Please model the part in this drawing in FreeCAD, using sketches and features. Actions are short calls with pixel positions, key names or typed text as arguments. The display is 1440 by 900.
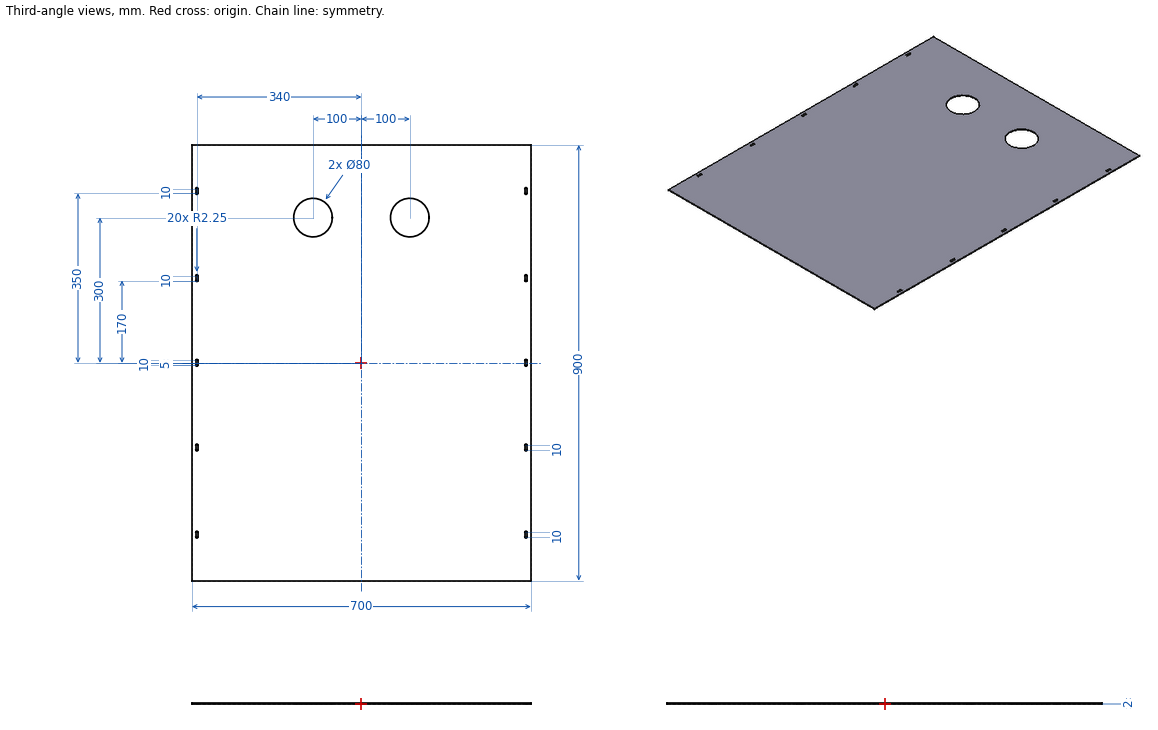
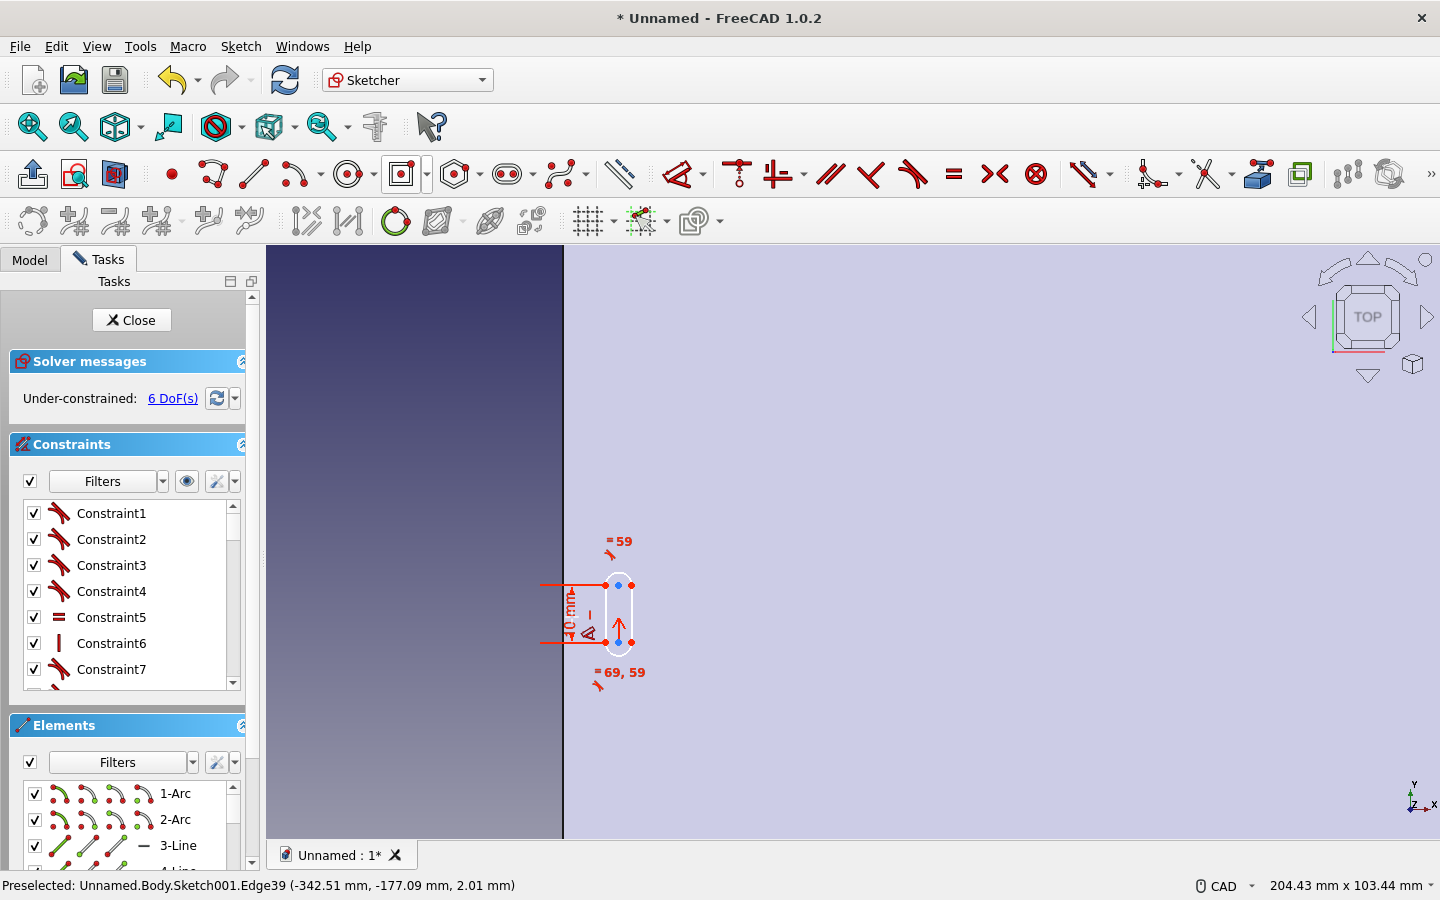
scroll(606, 635, down, 12)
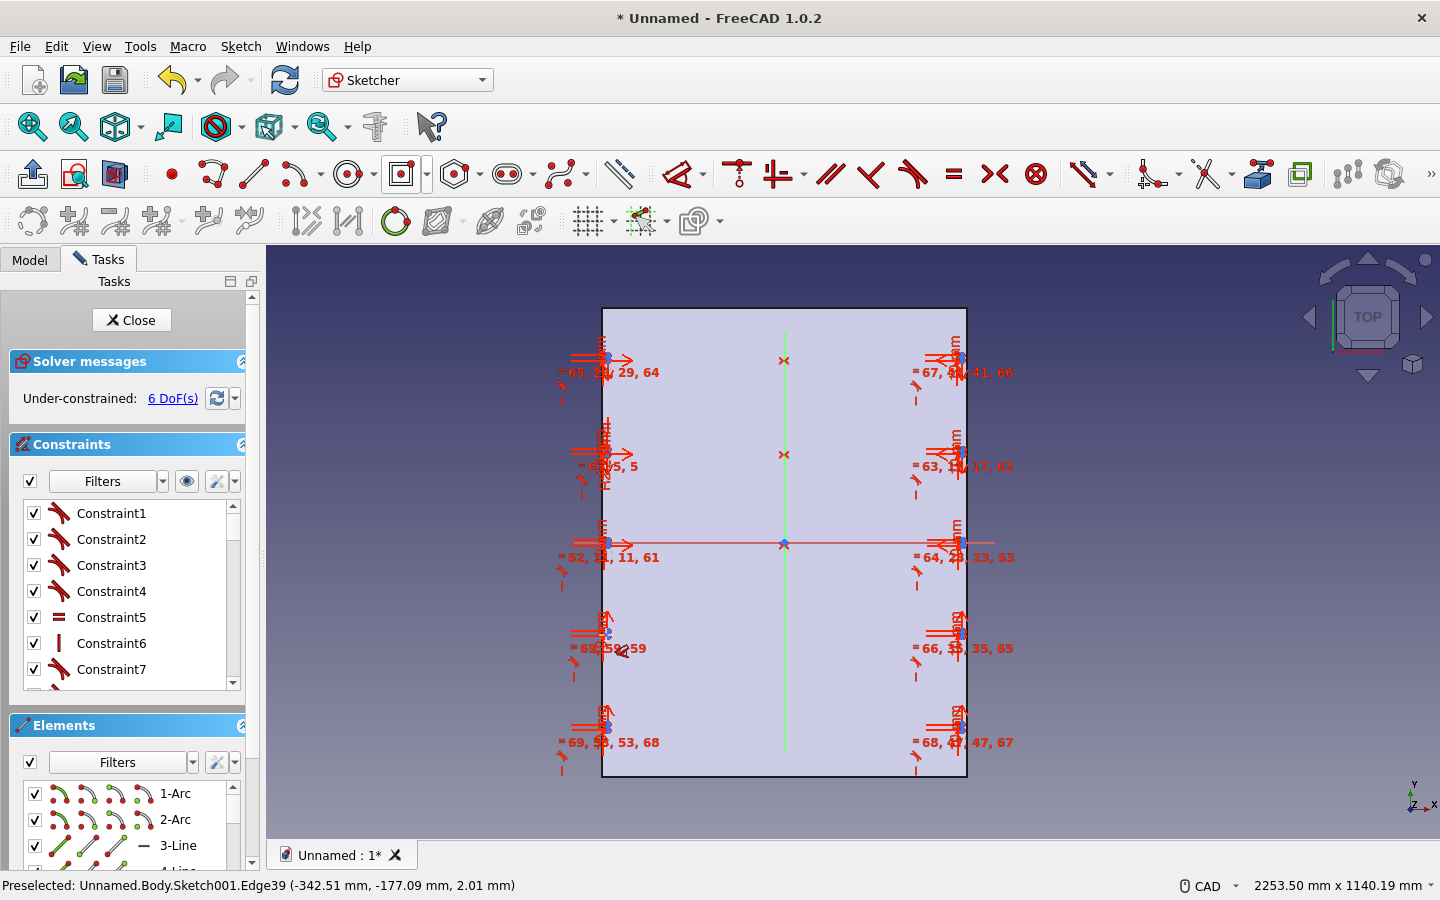
scroll(606, 546, up, 14)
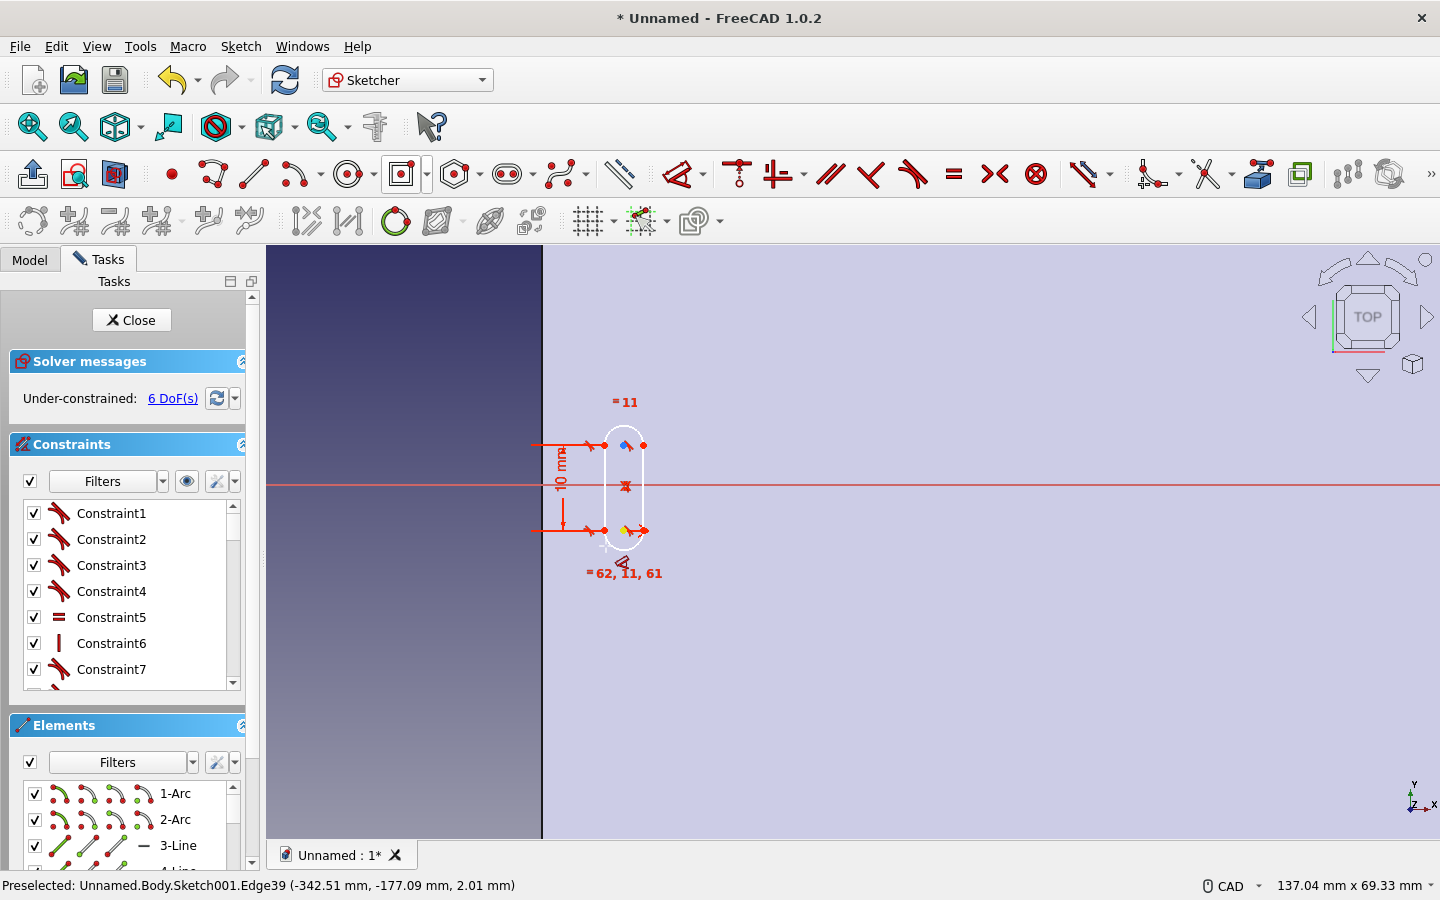
click(605, 531)
click(571, 508)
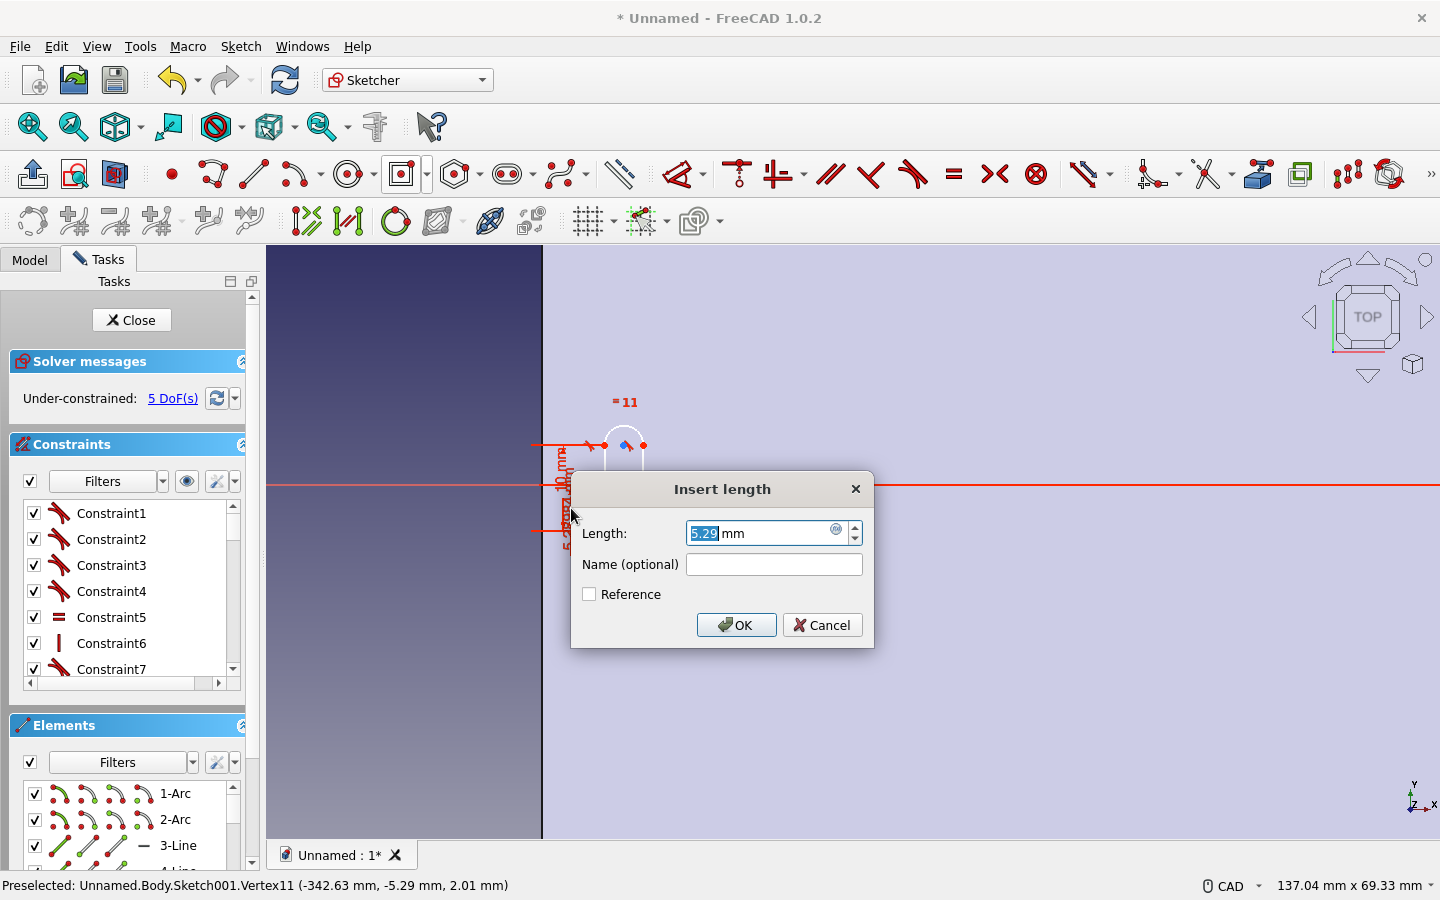
text(5)
key(Return)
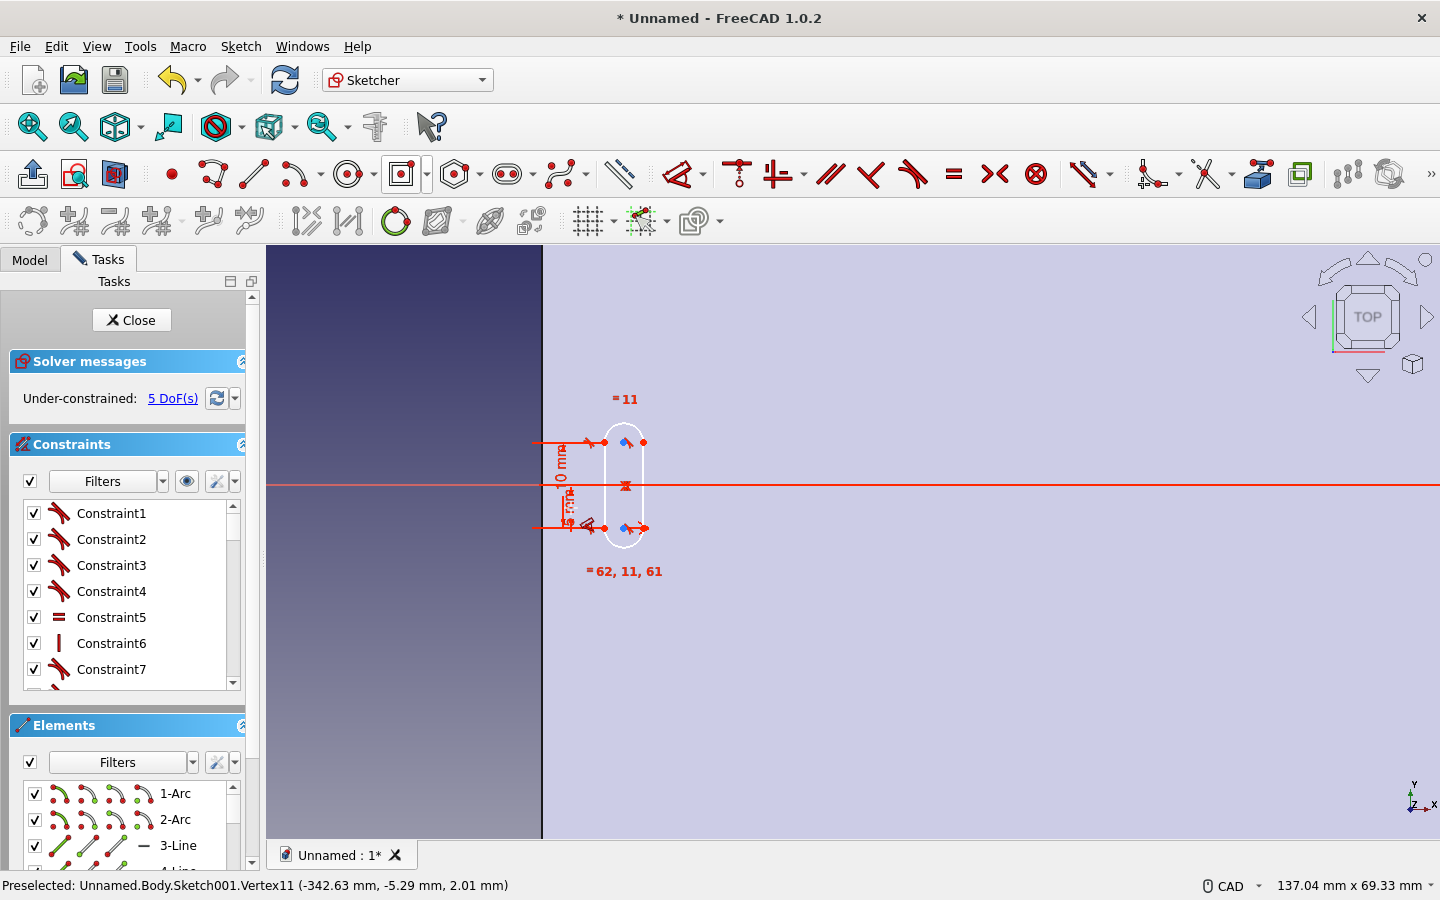
scroll(606, 546, down, 14)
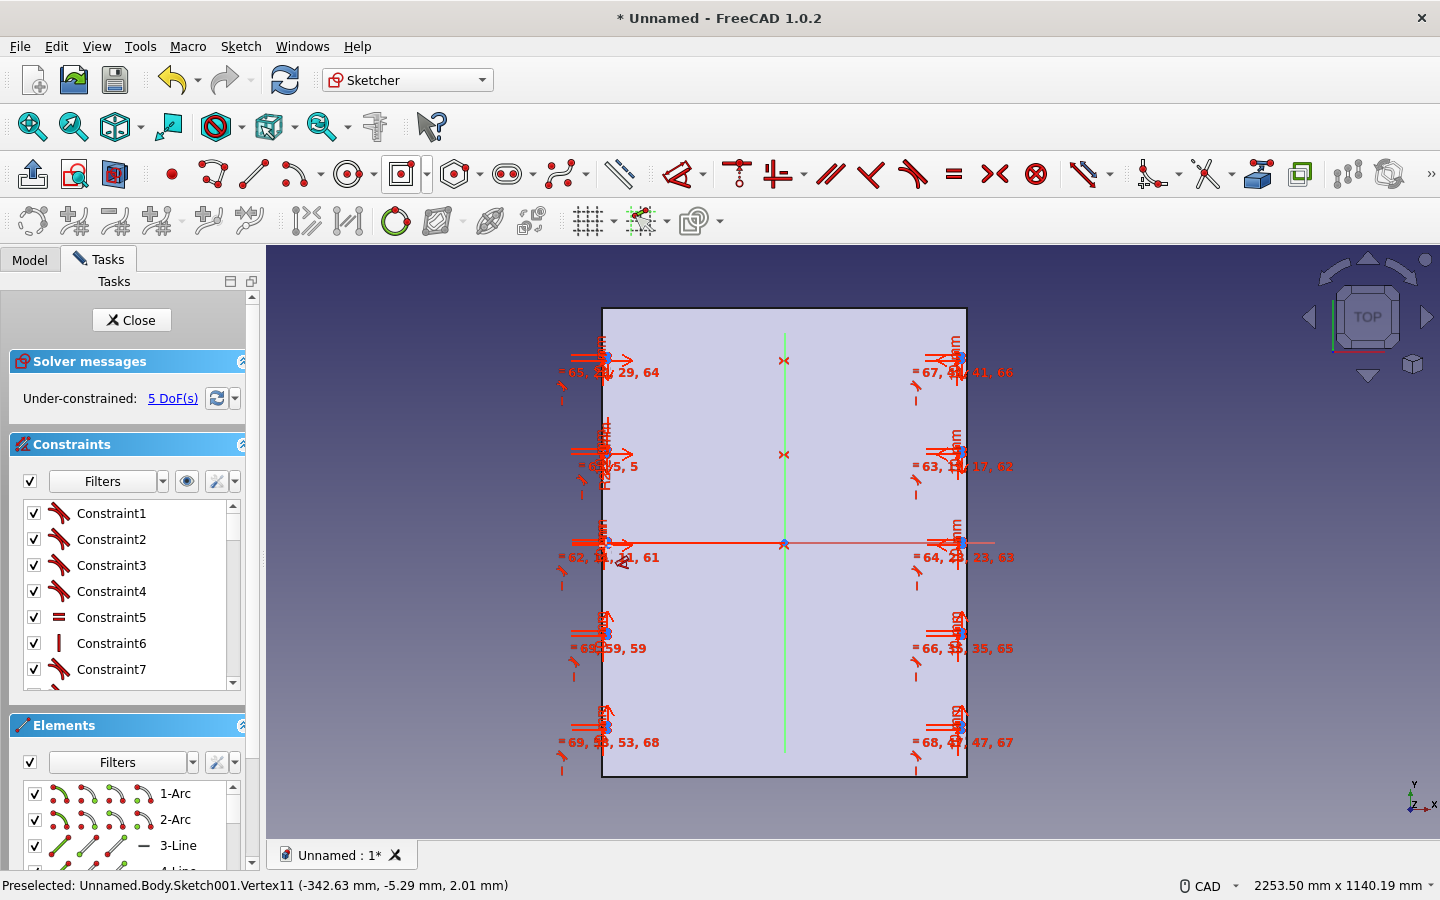
scroll(606, 454, up, 12)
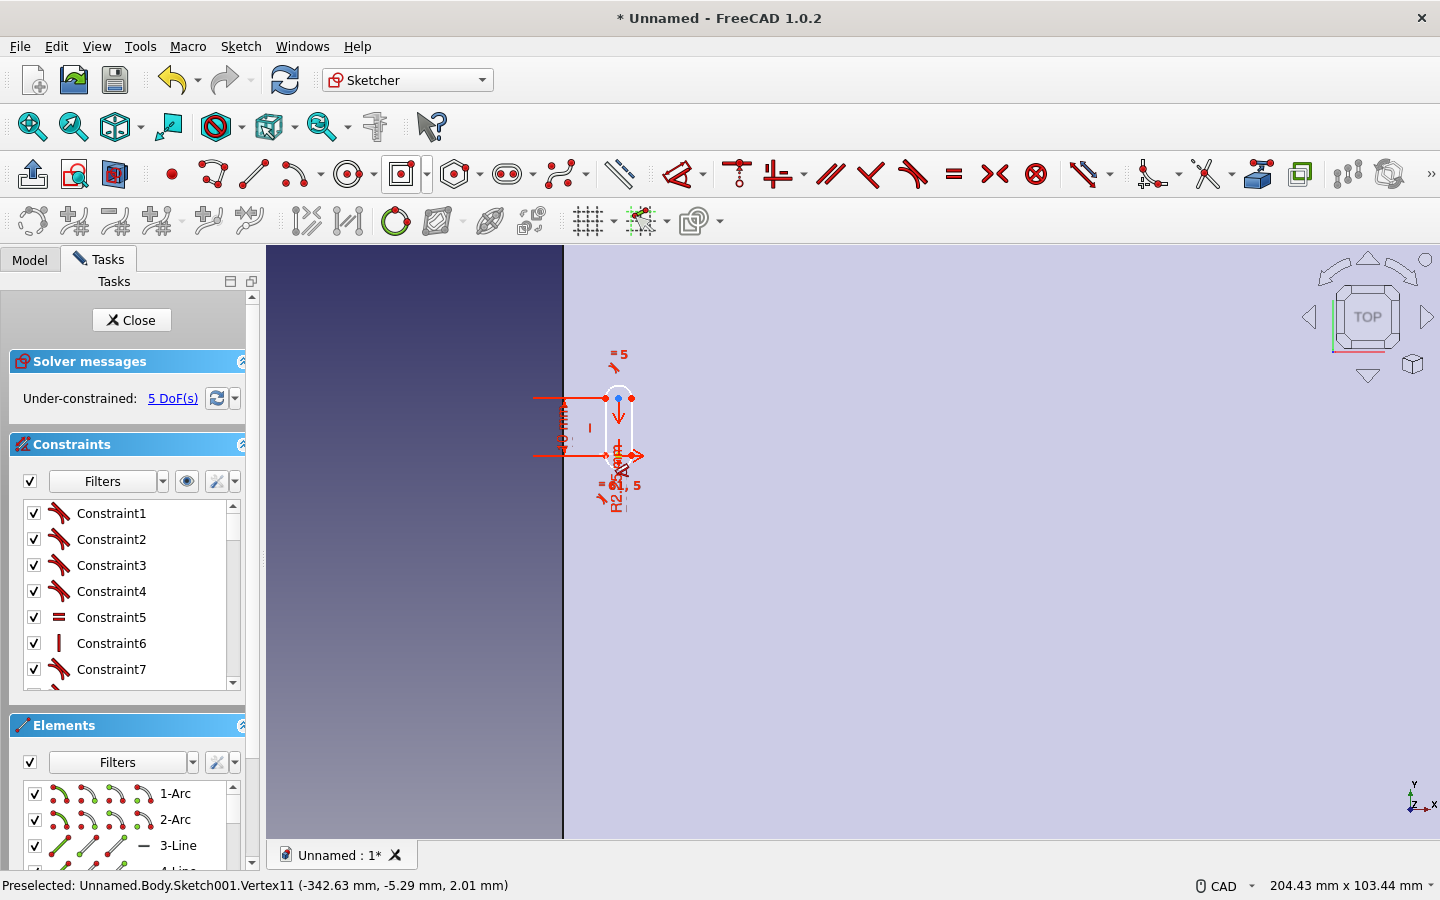
click(606, 456)
click(572, 633)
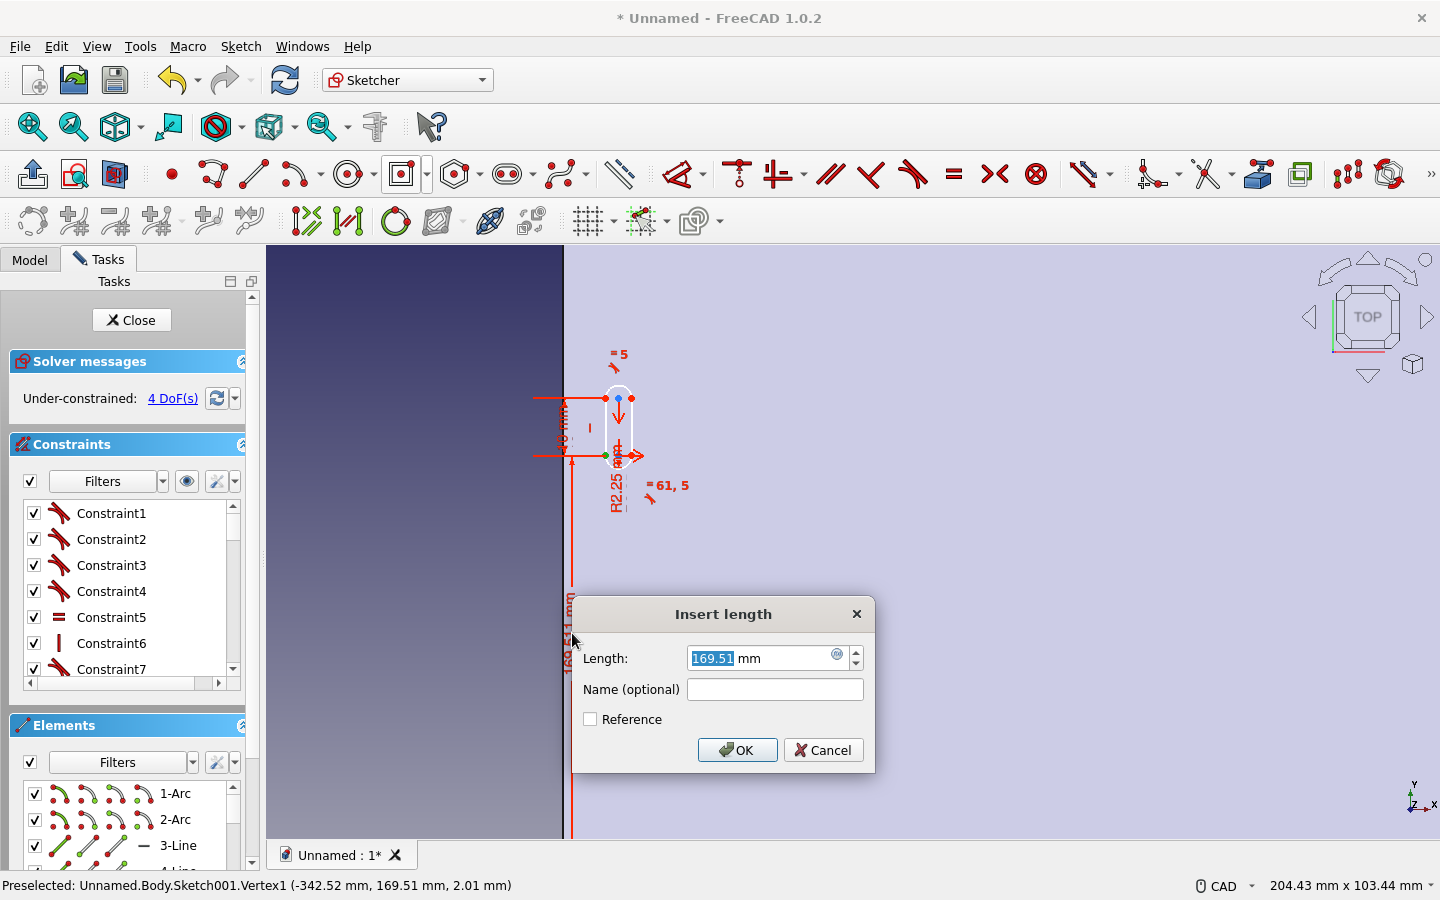
text(170)
key(Return)